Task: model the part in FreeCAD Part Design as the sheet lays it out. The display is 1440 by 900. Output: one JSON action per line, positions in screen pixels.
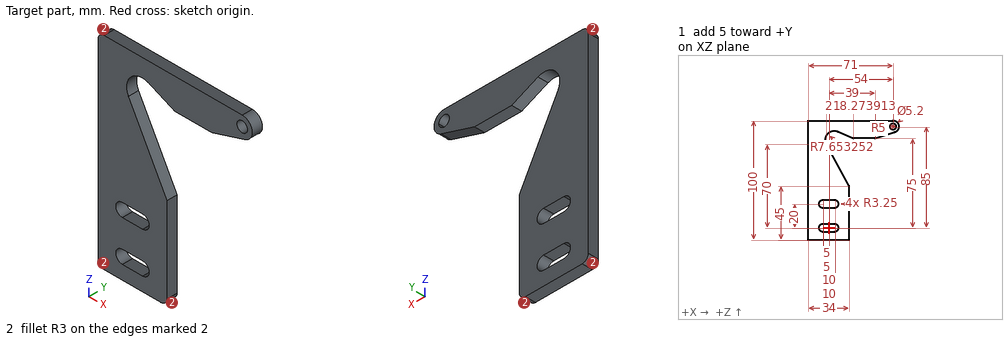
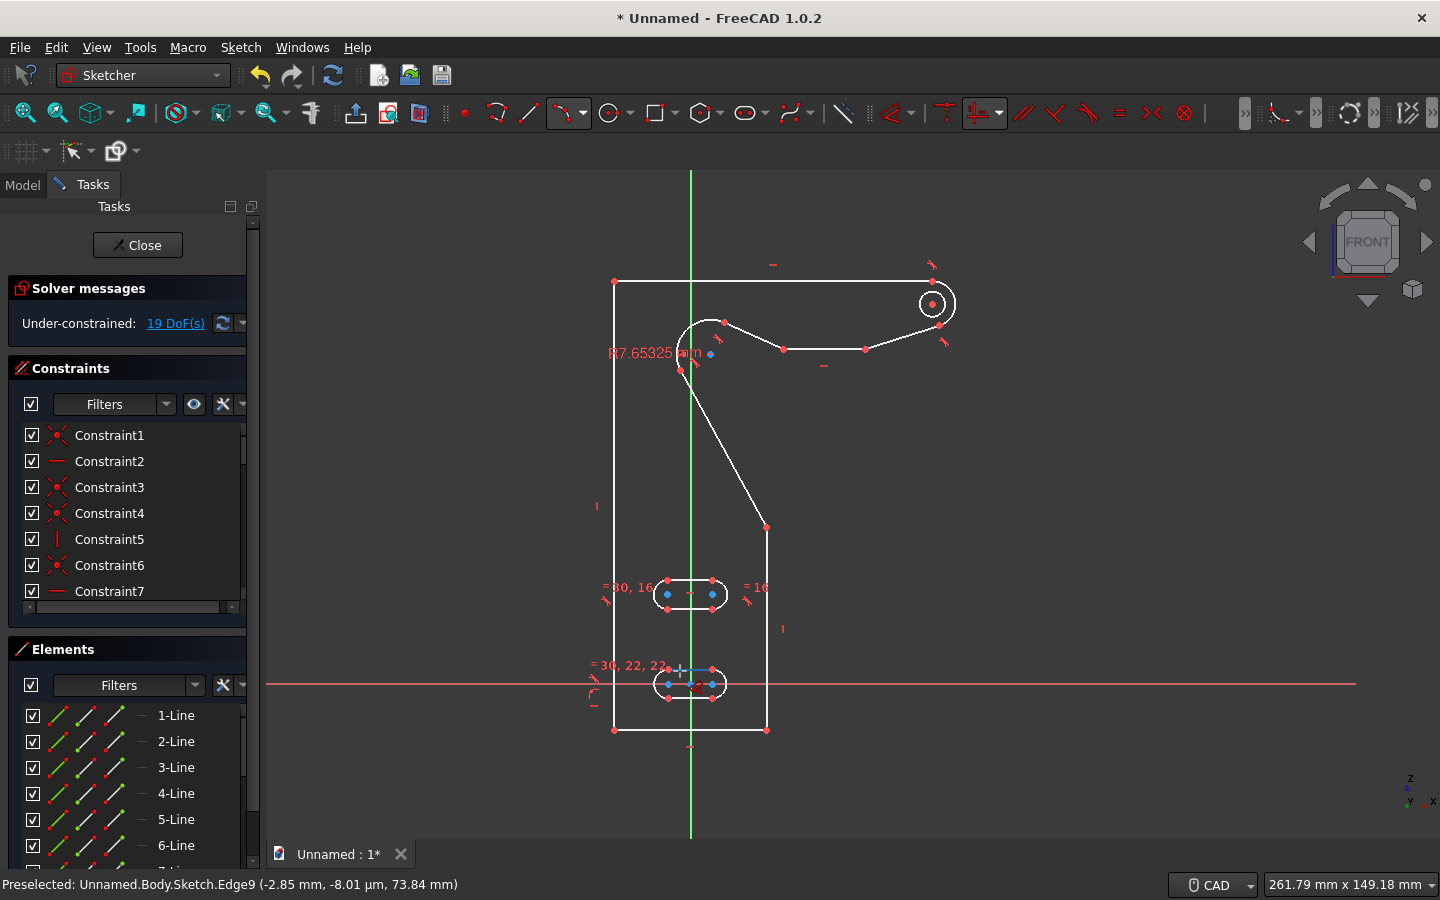
{"action": "scroll", "coordinate": [953, 313], "scroll_direction": "up", "scroll_amount": 3}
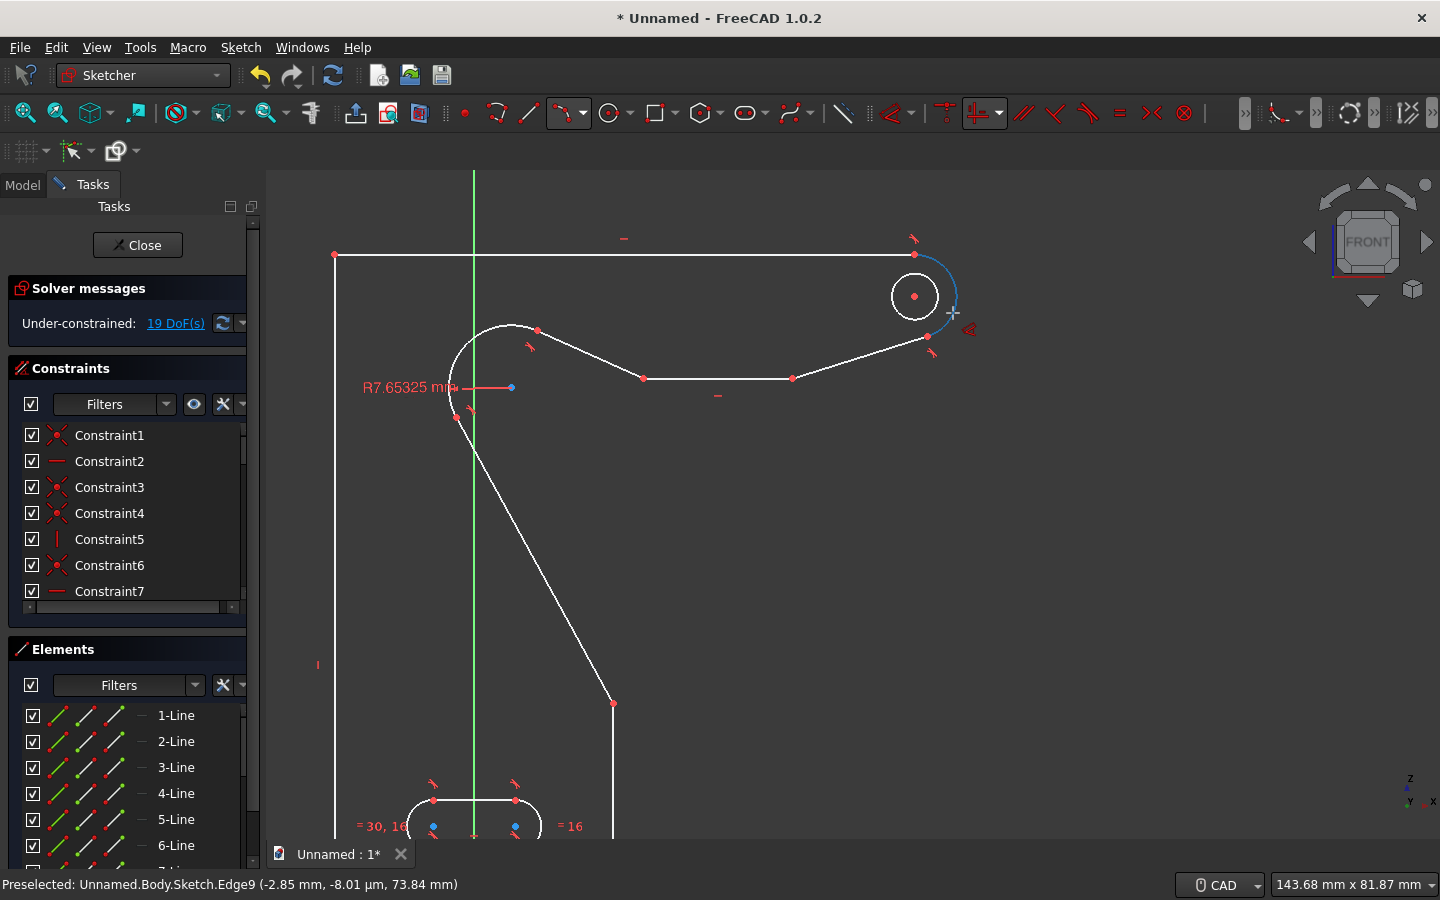
{"action": "left_click", "coordinate": [953, 313]}
{"action": "left_click", "coordinate": [982, 326]}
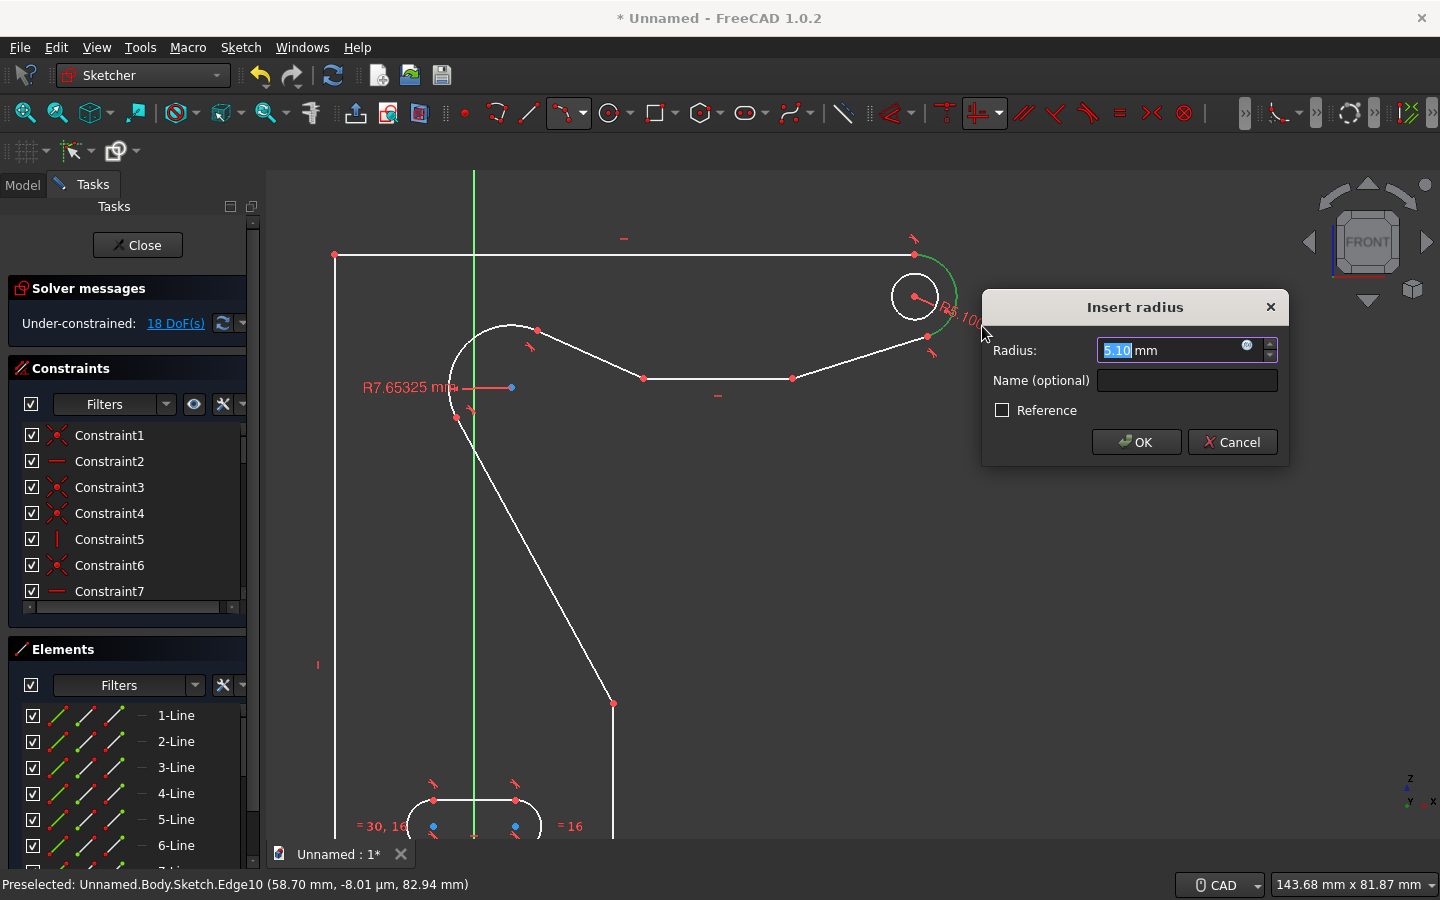
{"action": "type", "text": "5"}
{"action": "key", "text": "Return"}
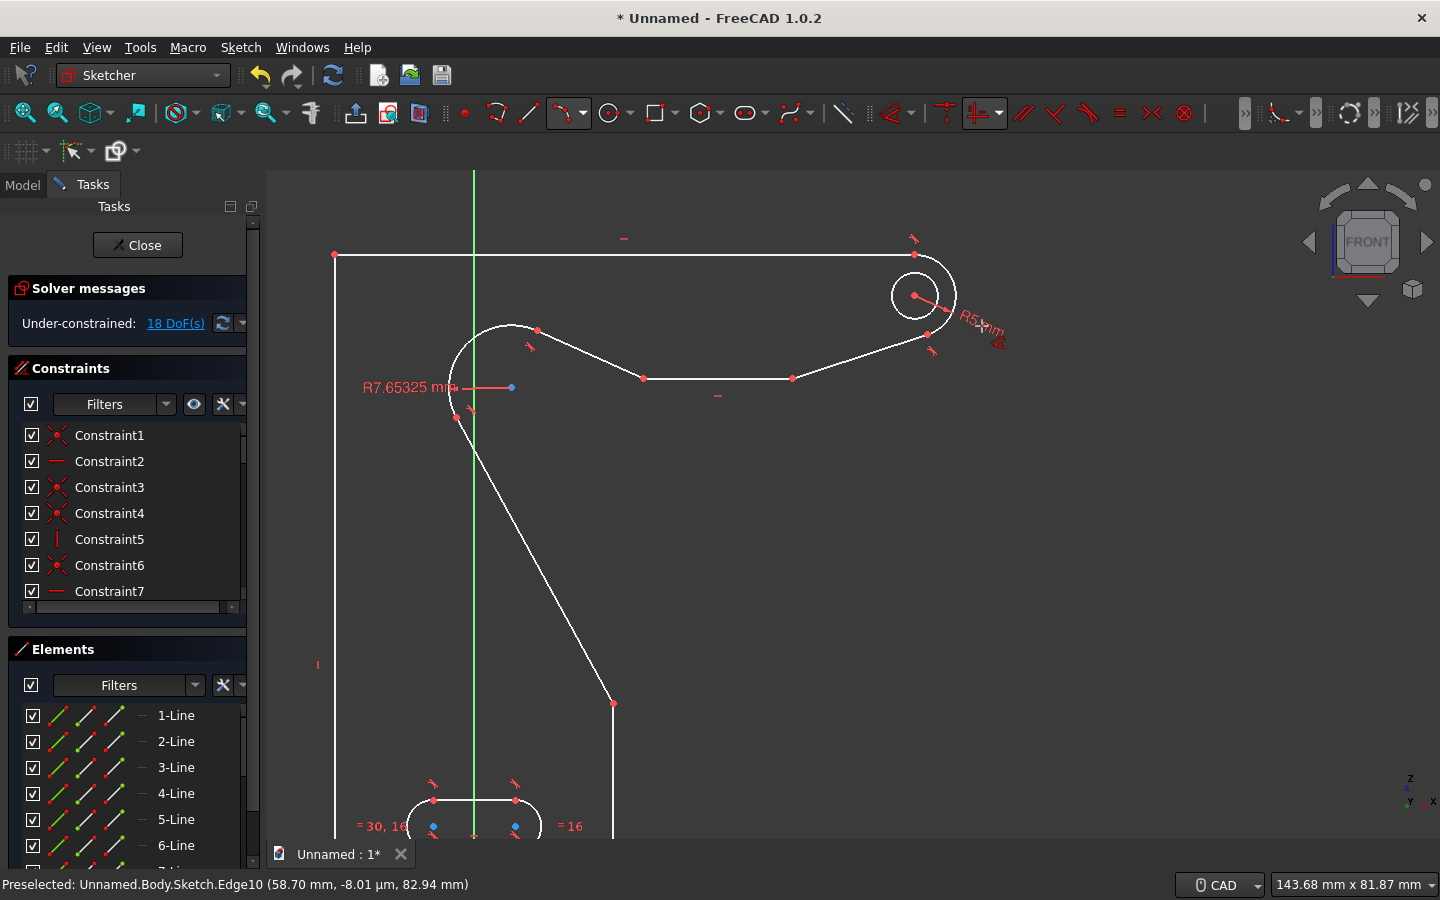
{"action": "scroll", "coordinate": [412, 811], "scroll_direction": "up", "scroll_amount": 3}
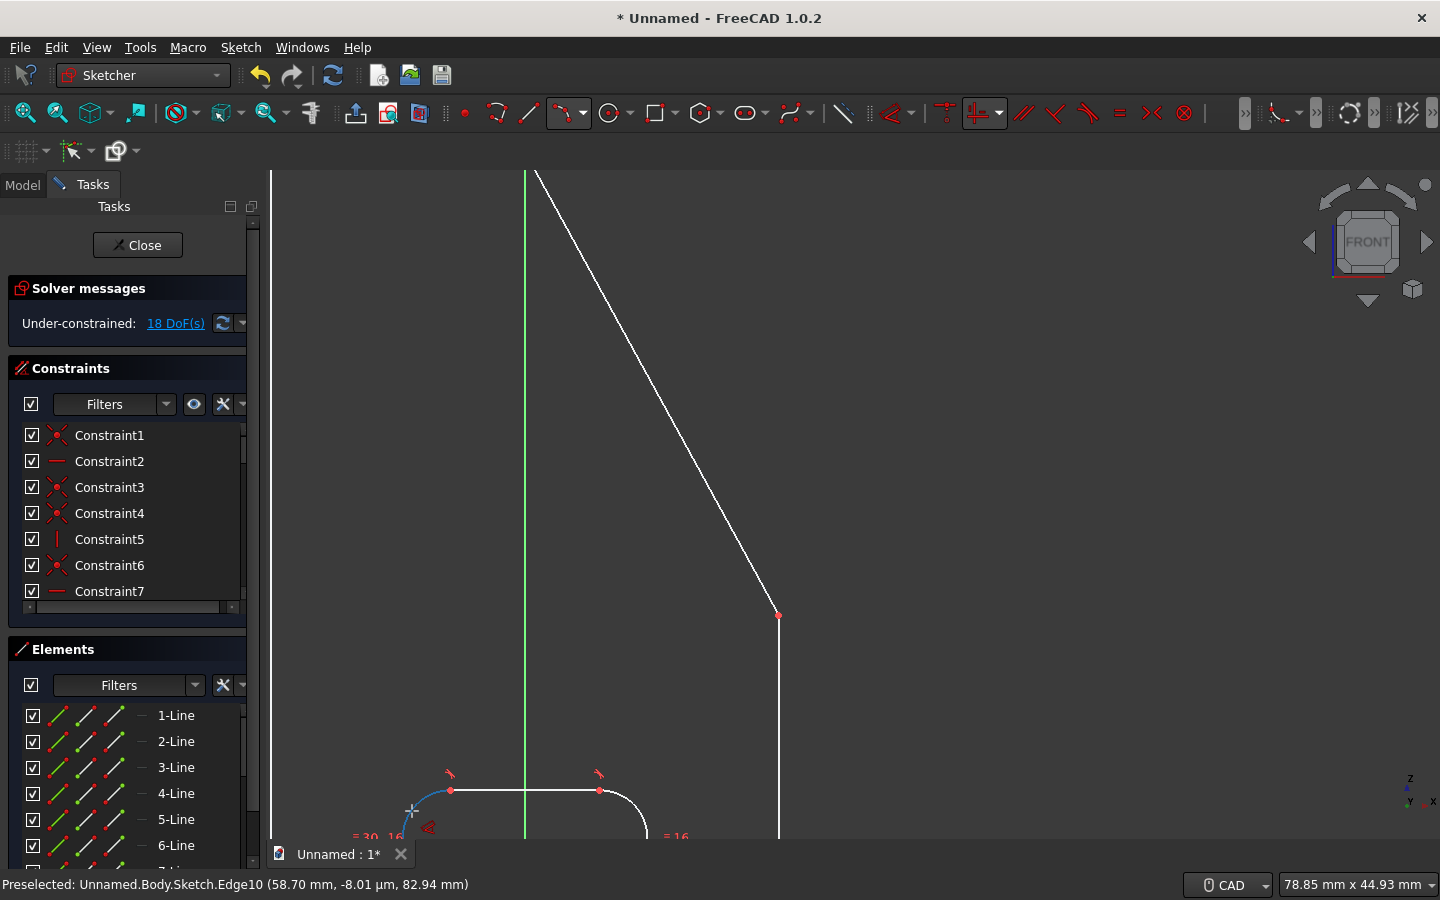
{"action": "left_click", "coordinate": [412, 810]}
{"action": "left_click", "coordinate": [386, 791]}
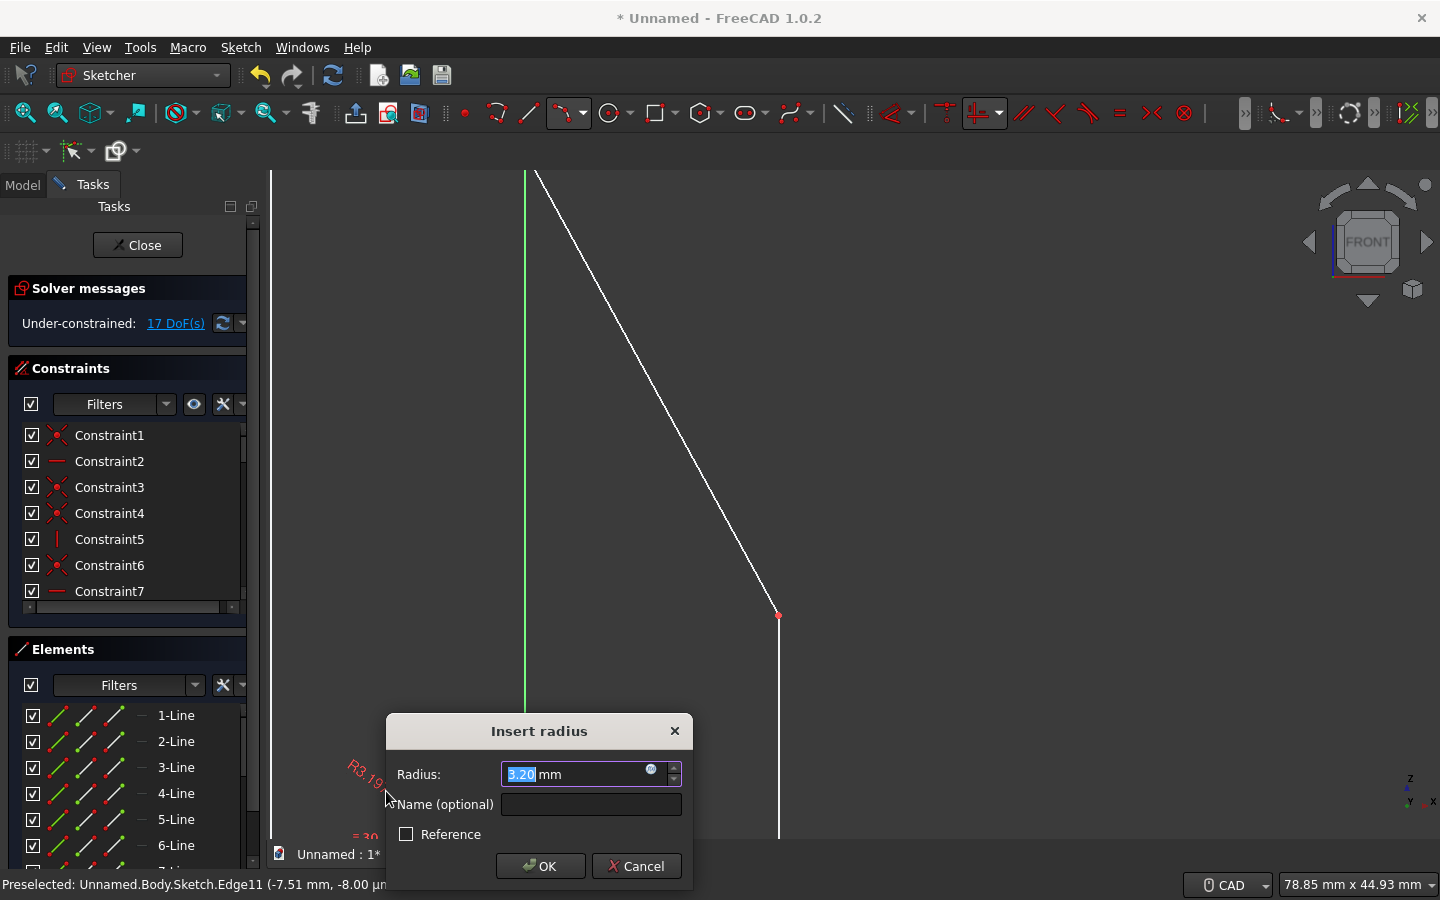
{"action": "type", "text": "3.25"}
{"action": "key", "text": "Return"}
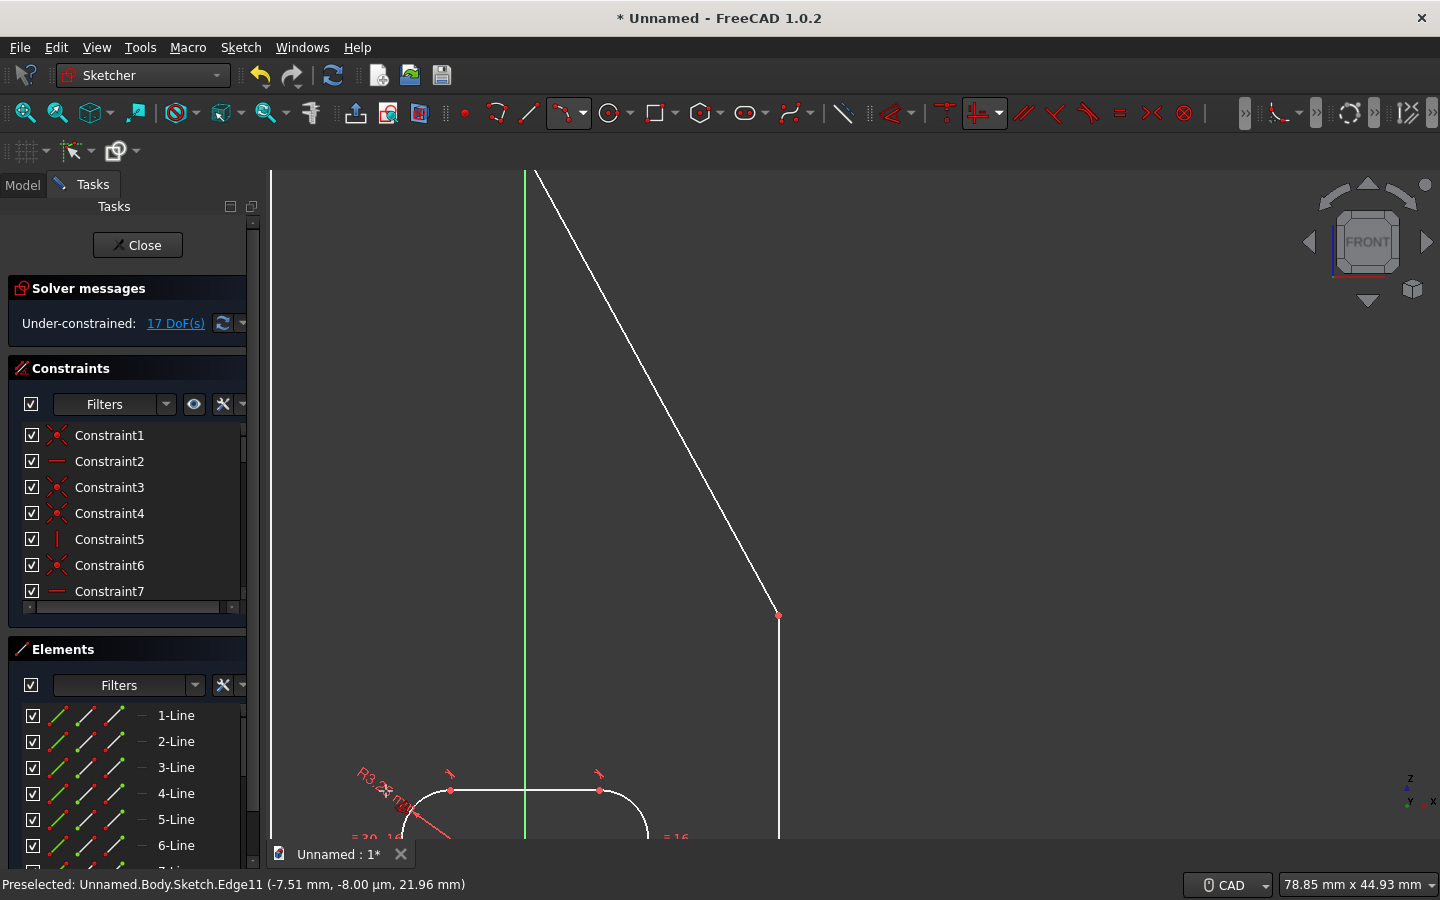
{"action": "scroll", "coordinate": [762, 490], "scroll_direction": "down", "scroll_amount": 6}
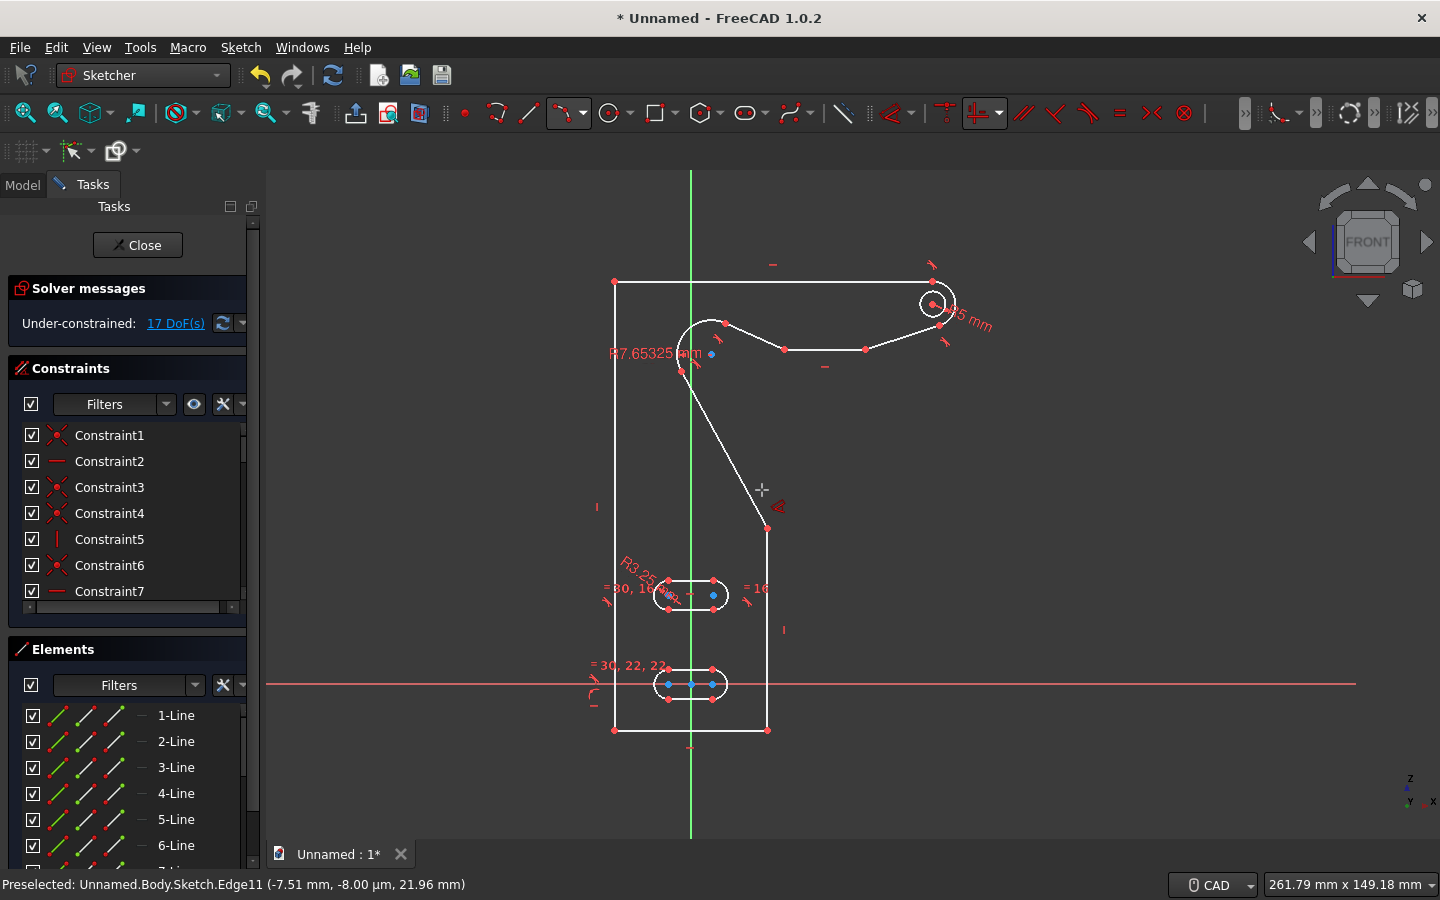
{"action": "scroll", "coordinate": [942, 295], "scroll_direction": "up", "scroll_amount": 3}